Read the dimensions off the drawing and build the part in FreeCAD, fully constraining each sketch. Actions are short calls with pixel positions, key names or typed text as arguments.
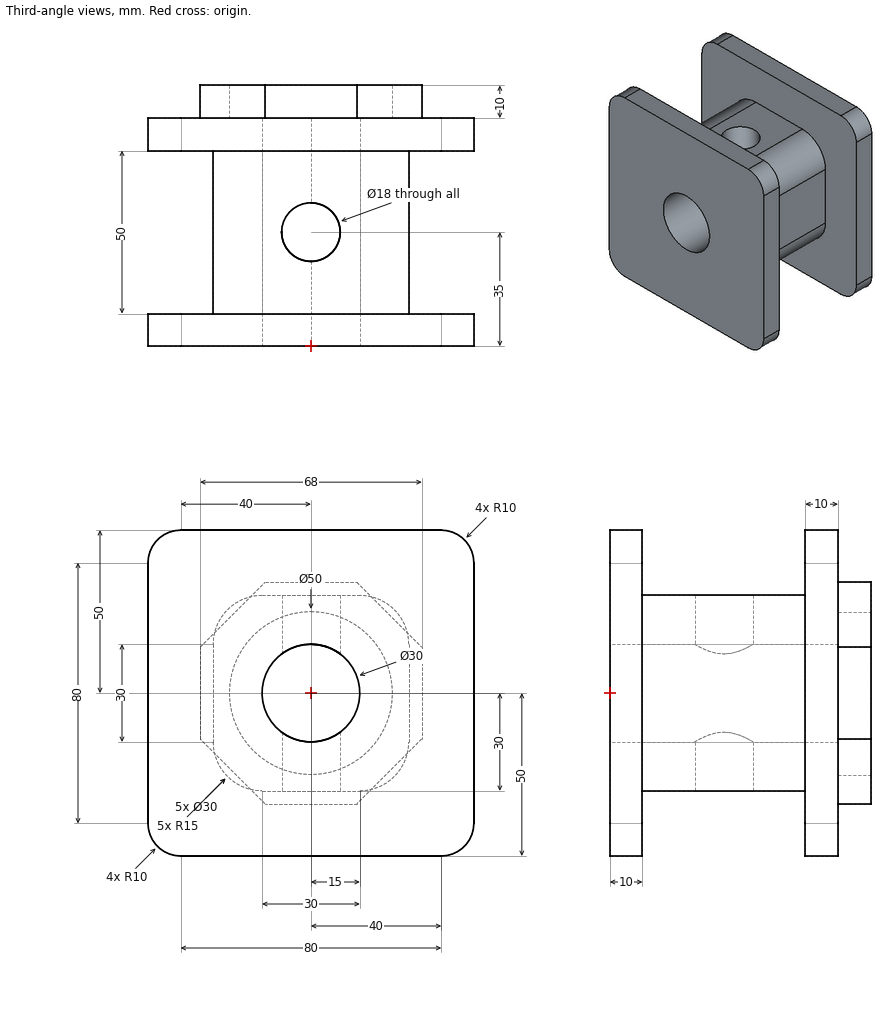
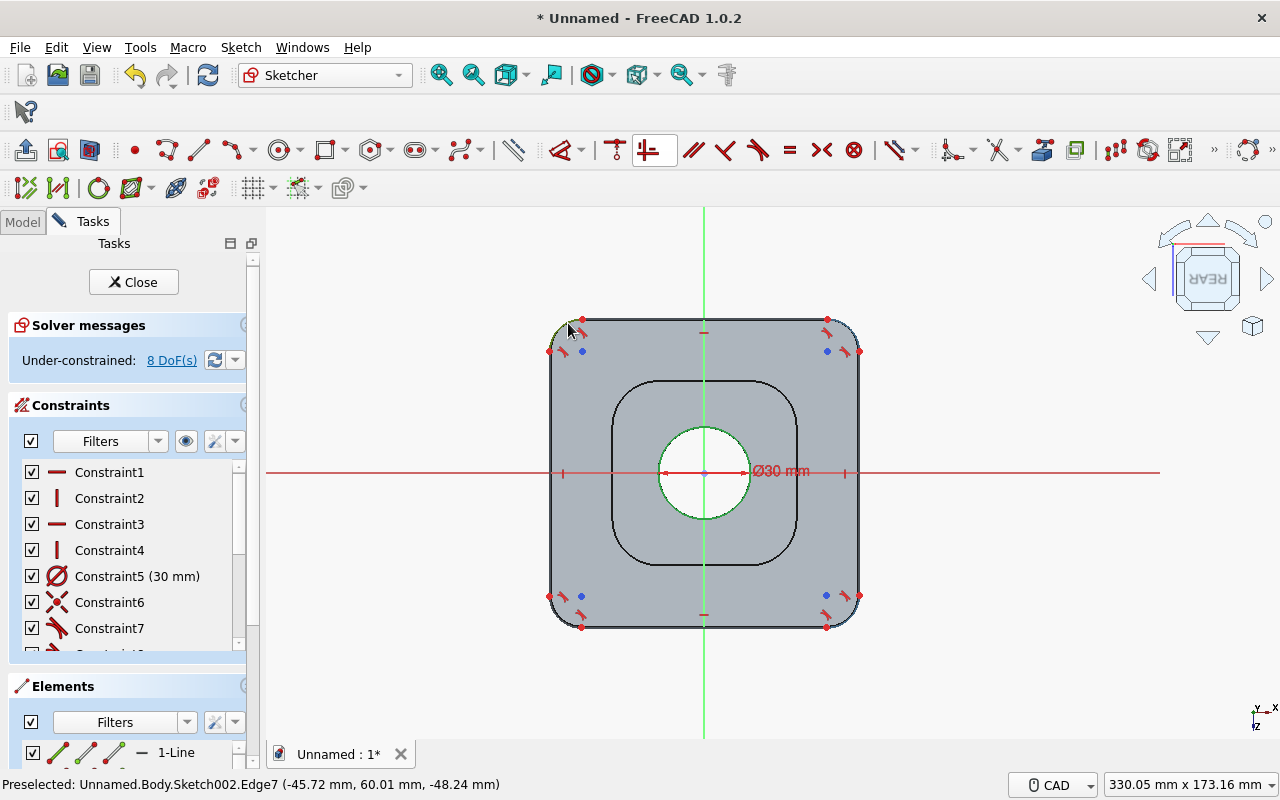
click(553, 610)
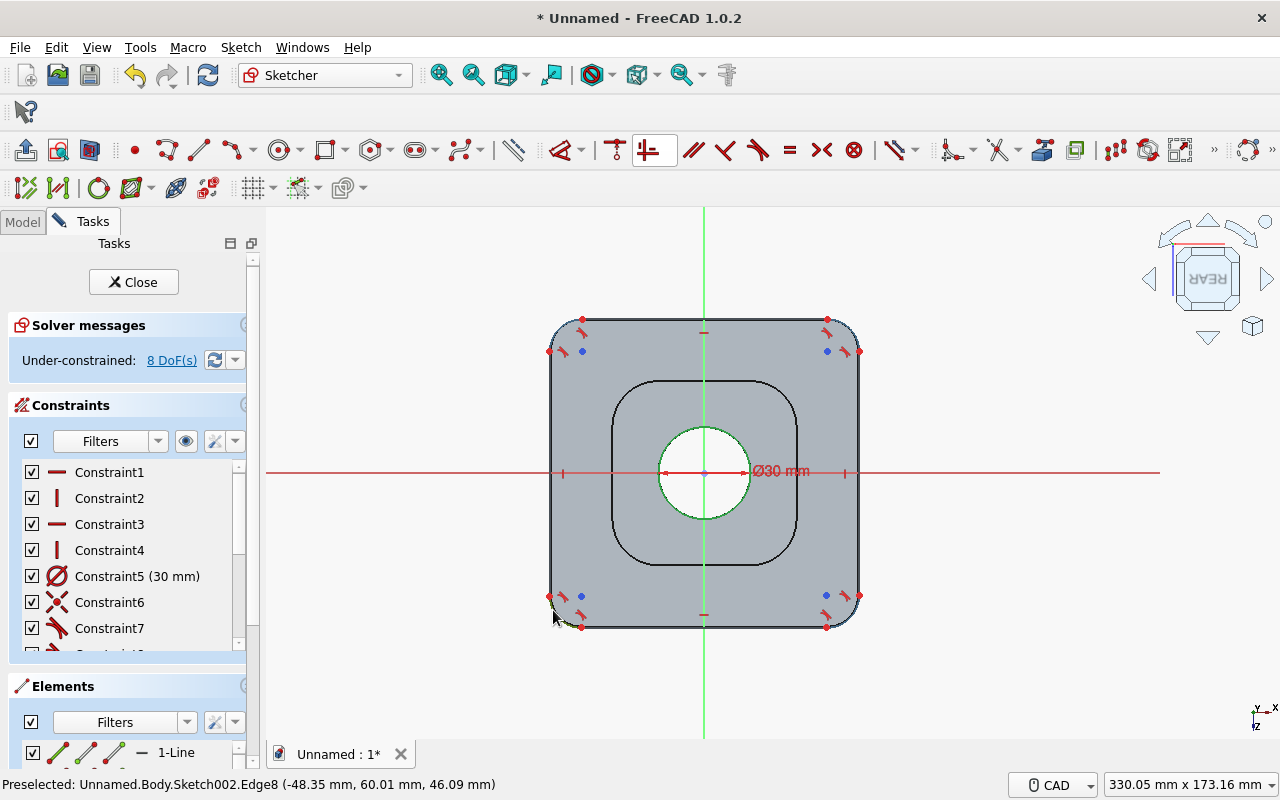
click(790, 150)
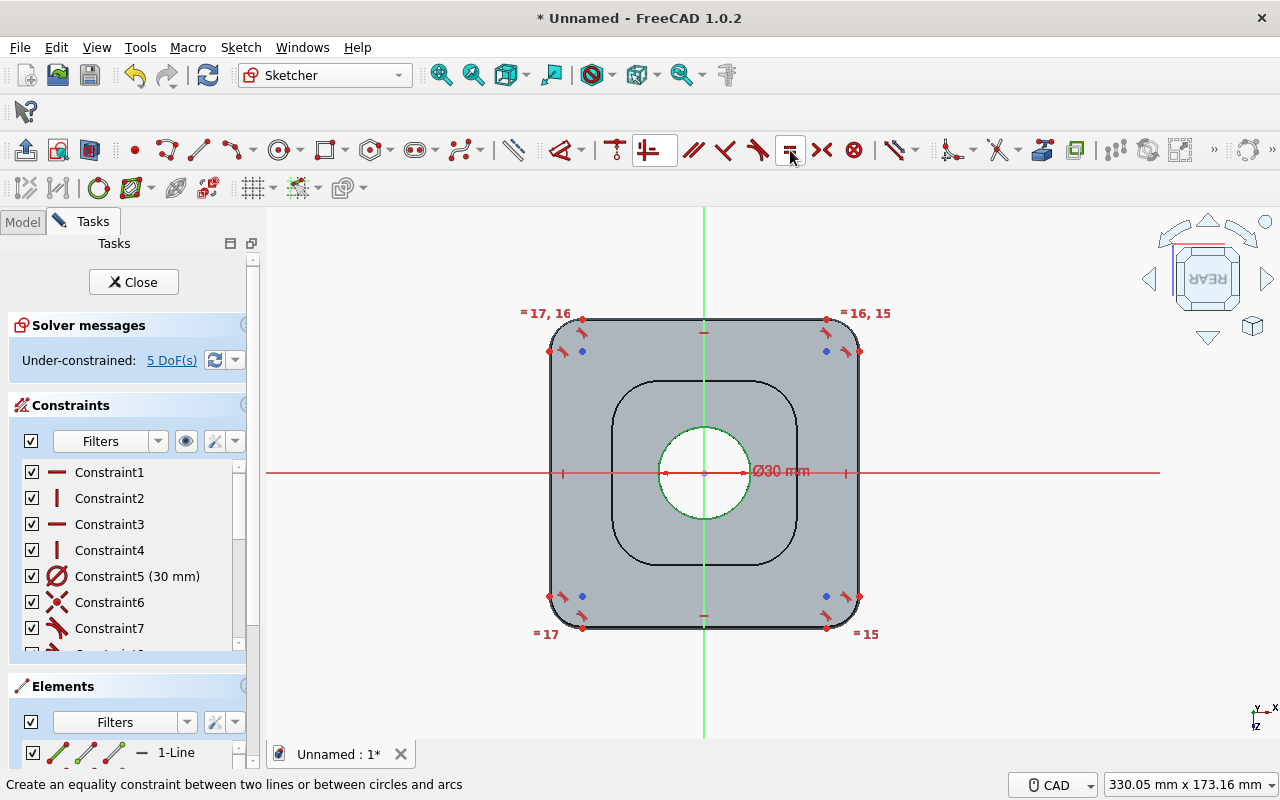
click(560, 150)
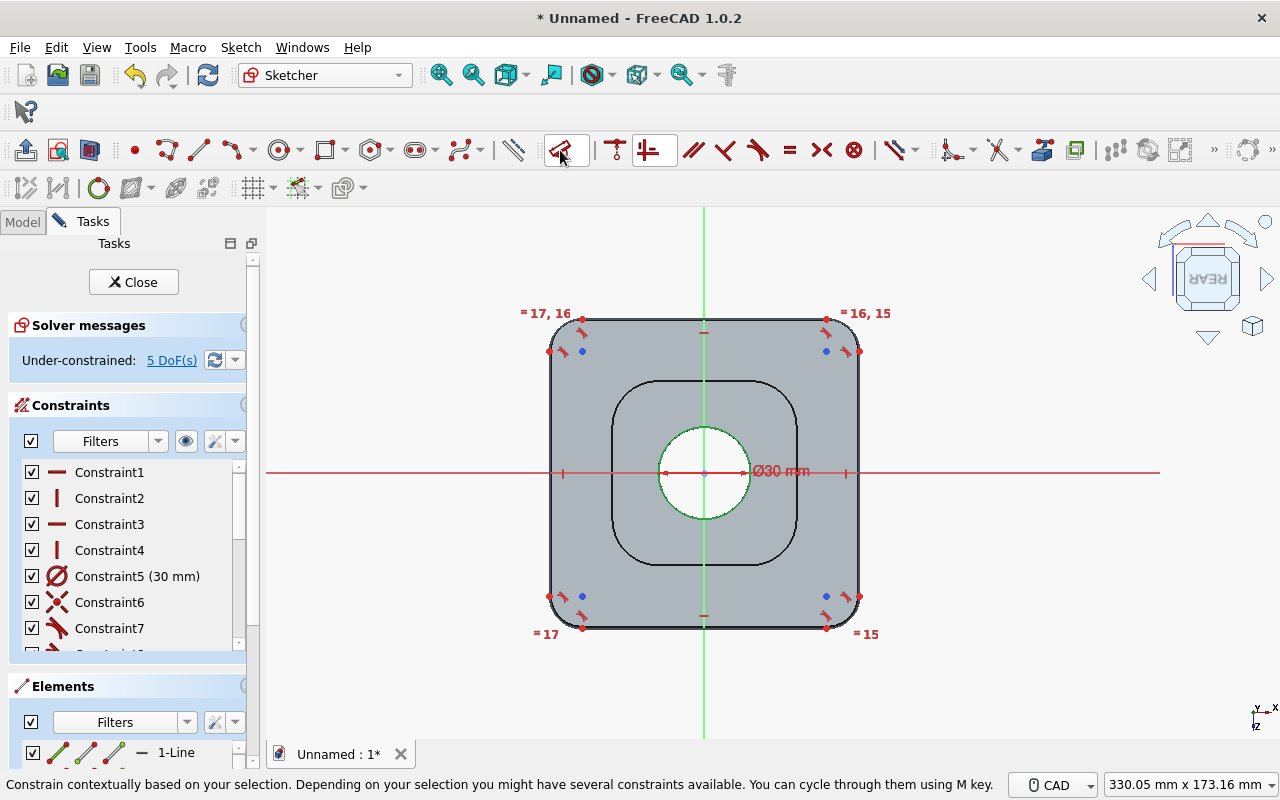
scroll(842, 625, up, 2)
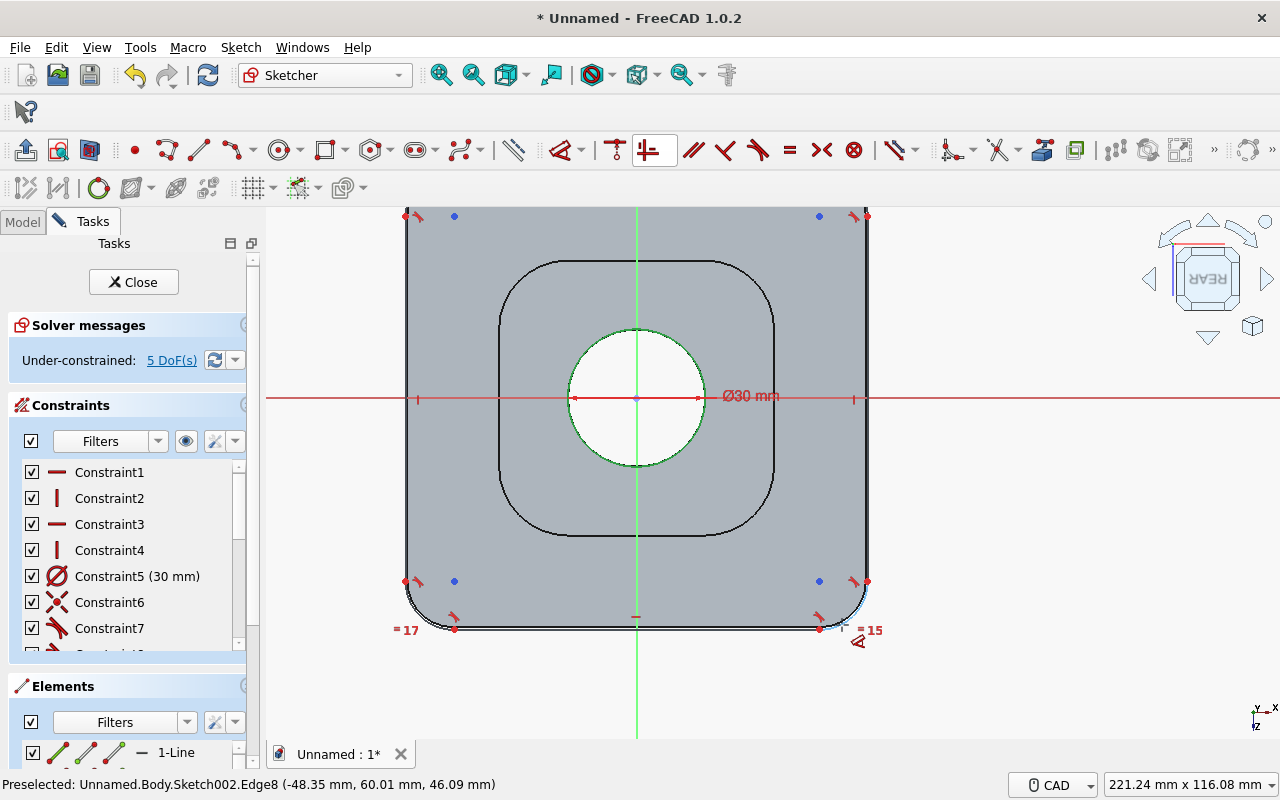
click(841, 625)
click(855, 654)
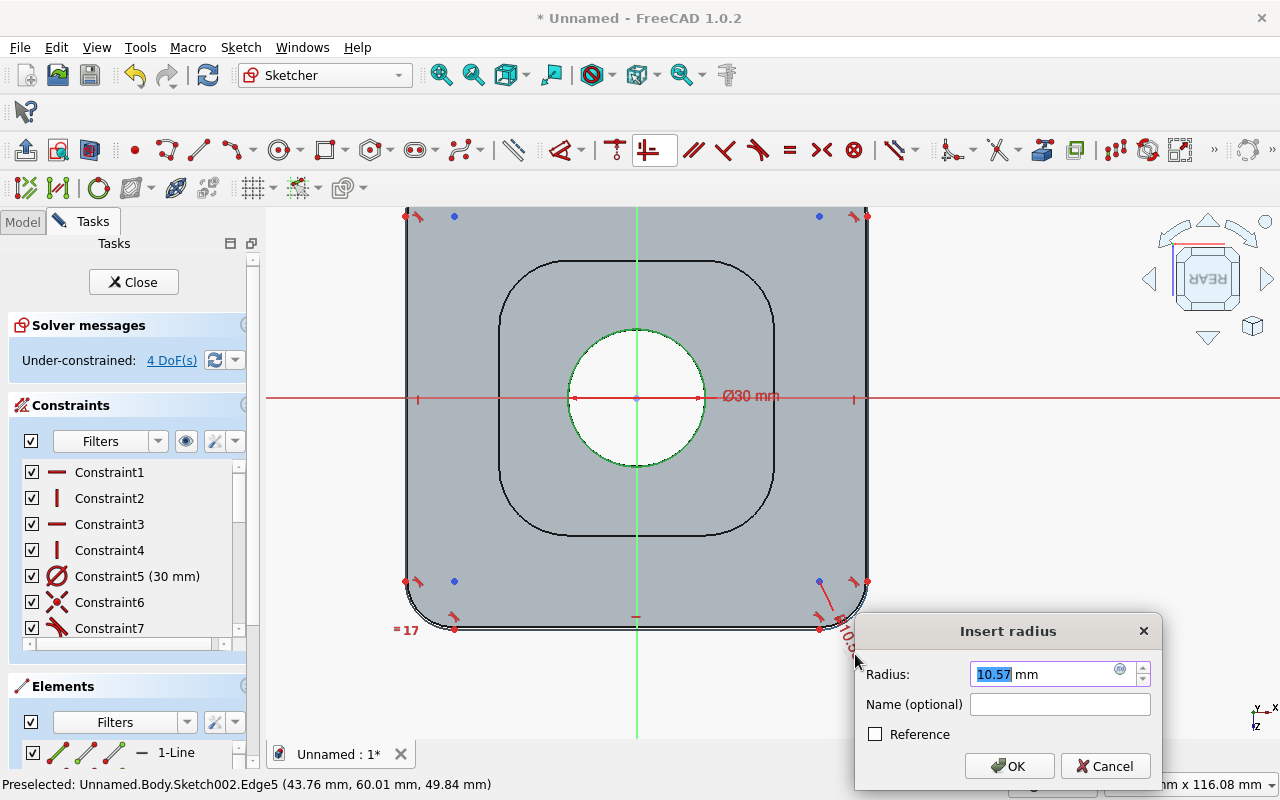
text(10)
key(Return)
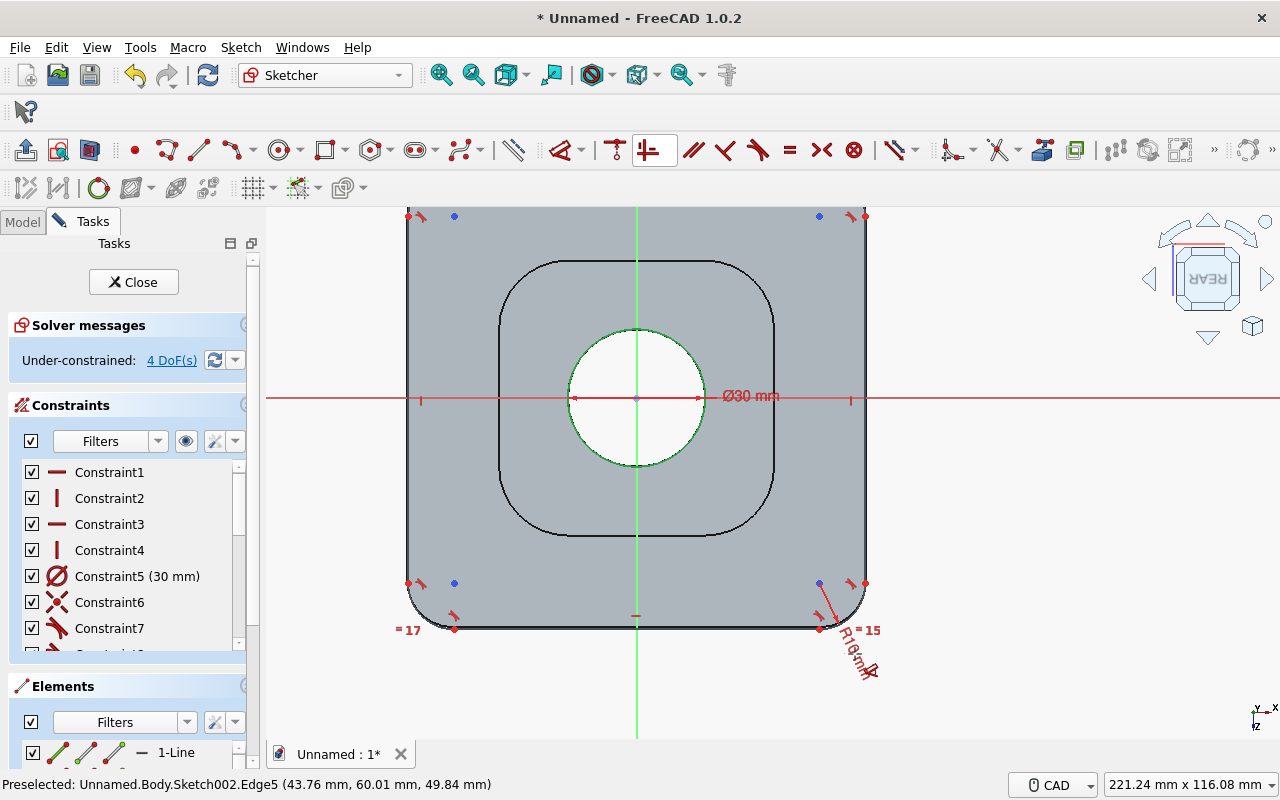
click(564, 629)
click(553, 663)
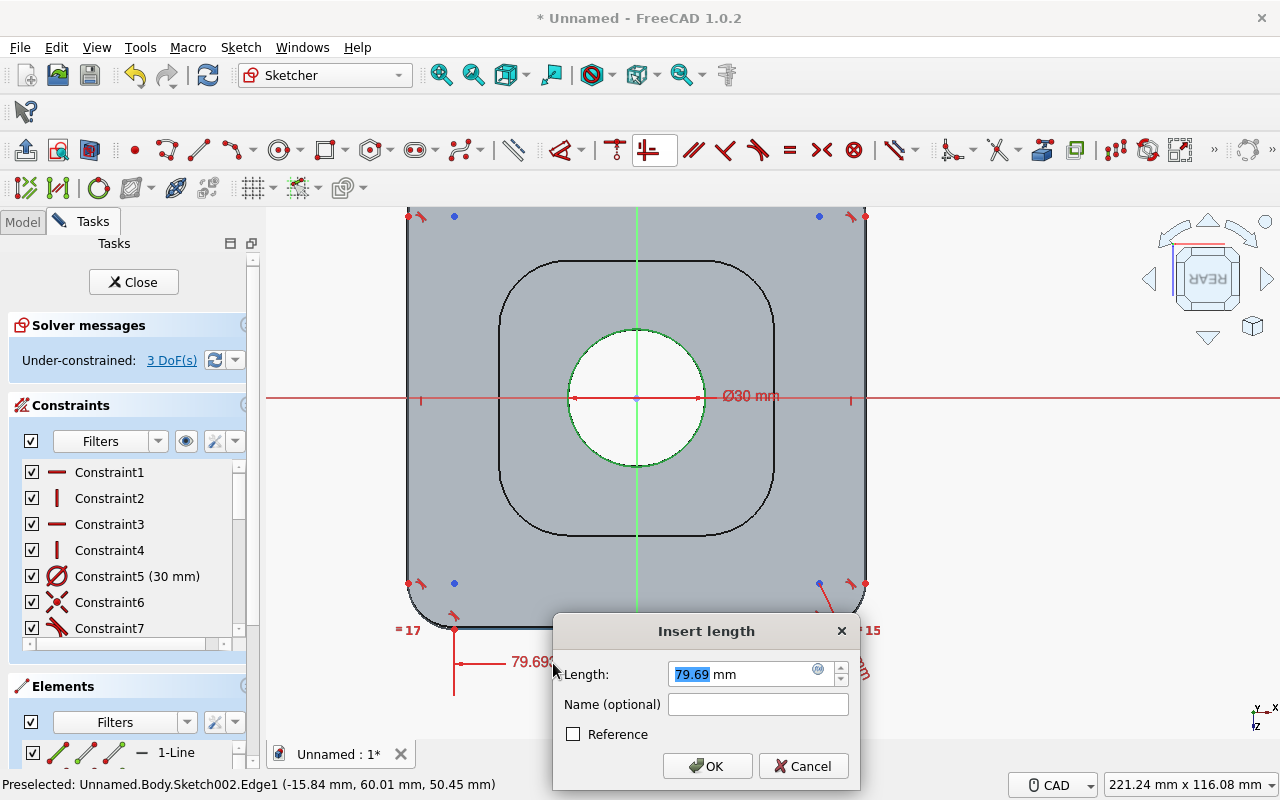
text(80)
key(Return)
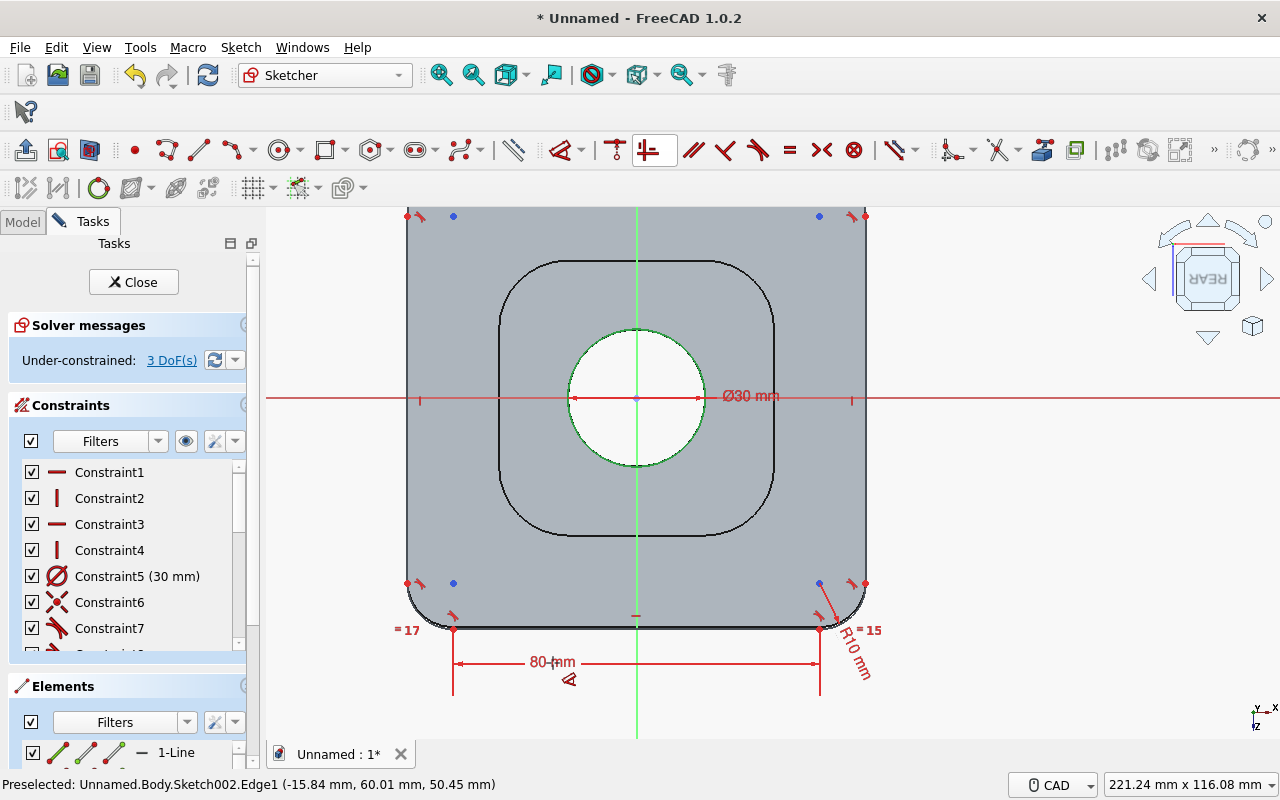
click(866, 473)
click(900, 329)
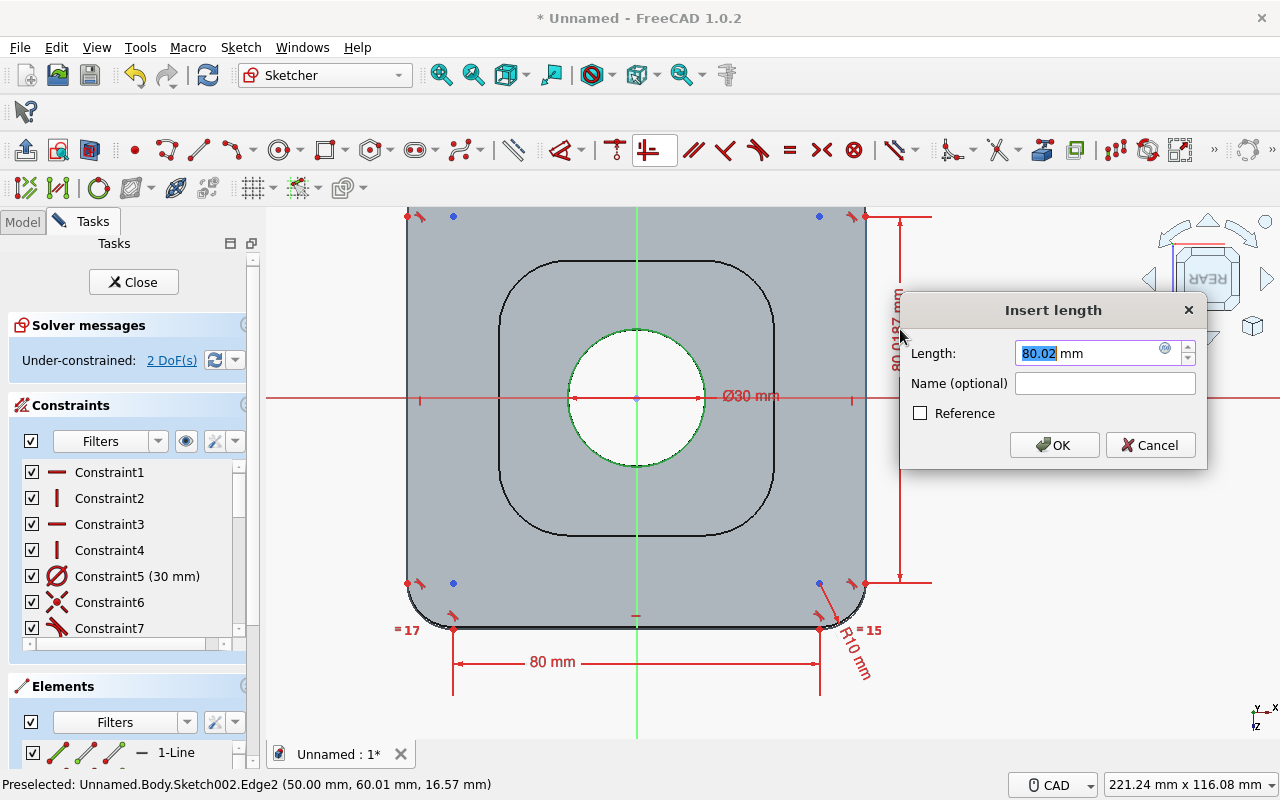
text(80)
key(Return)